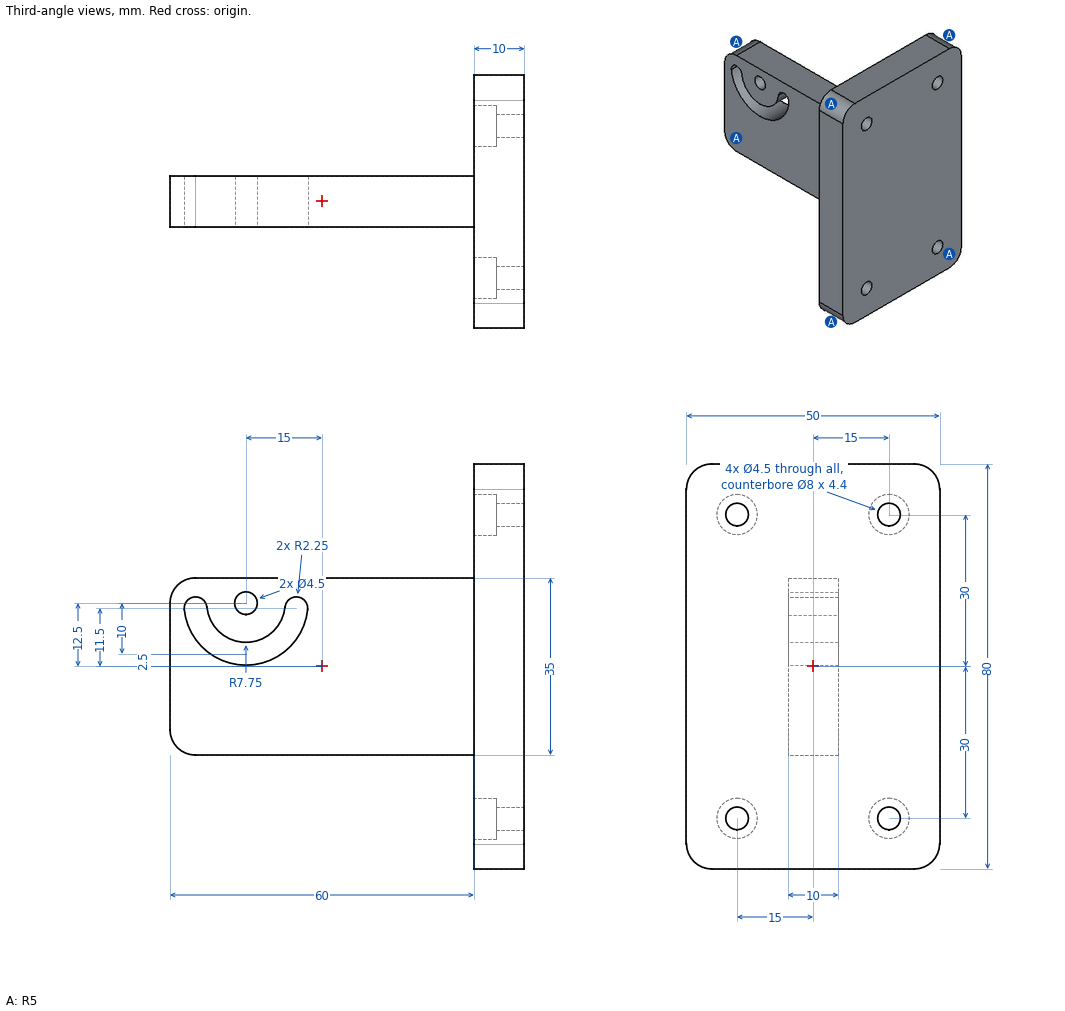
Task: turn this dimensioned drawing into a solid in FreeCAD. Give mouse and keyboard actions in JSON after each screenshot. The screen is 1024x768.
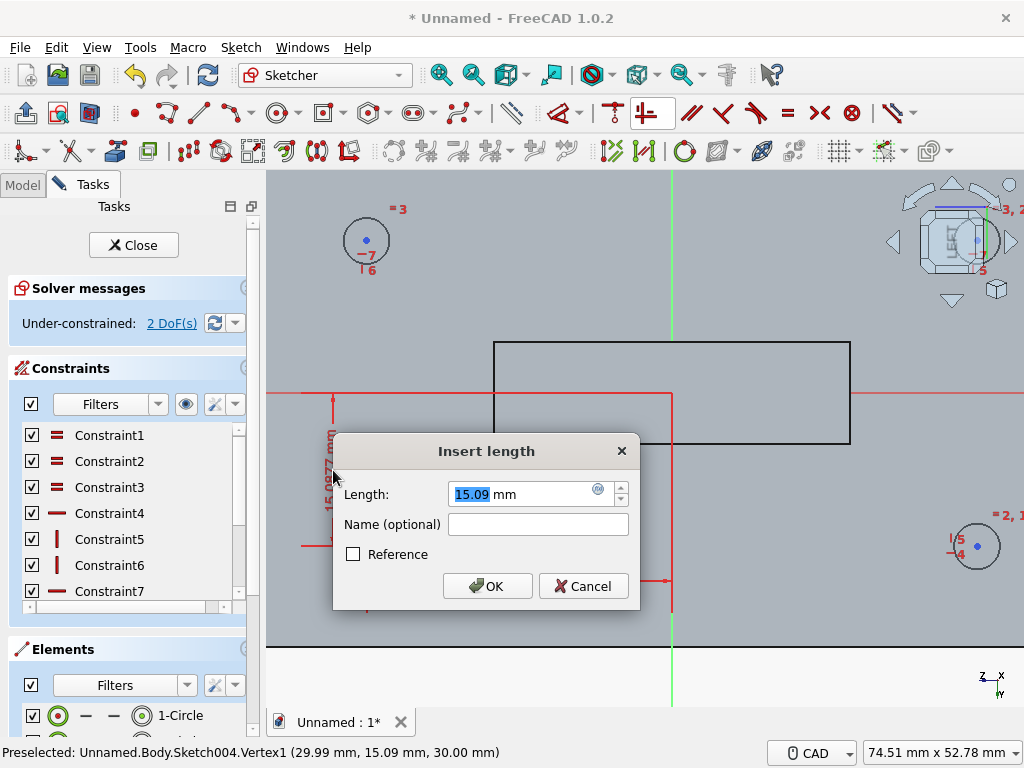
{"action": "type", "text": "15"}
{"action": "key", "text": "Return"}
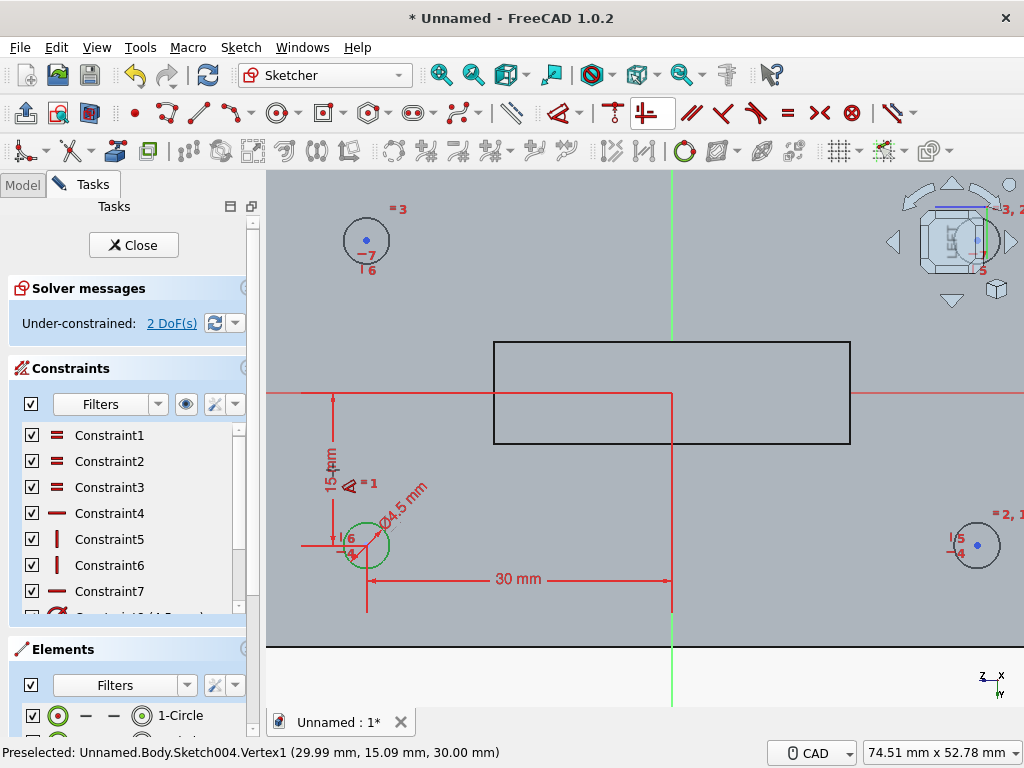
{"action": "scroll", "coordinate": [383, 531], "scroll_direction": "down", "scroll_amount": 2}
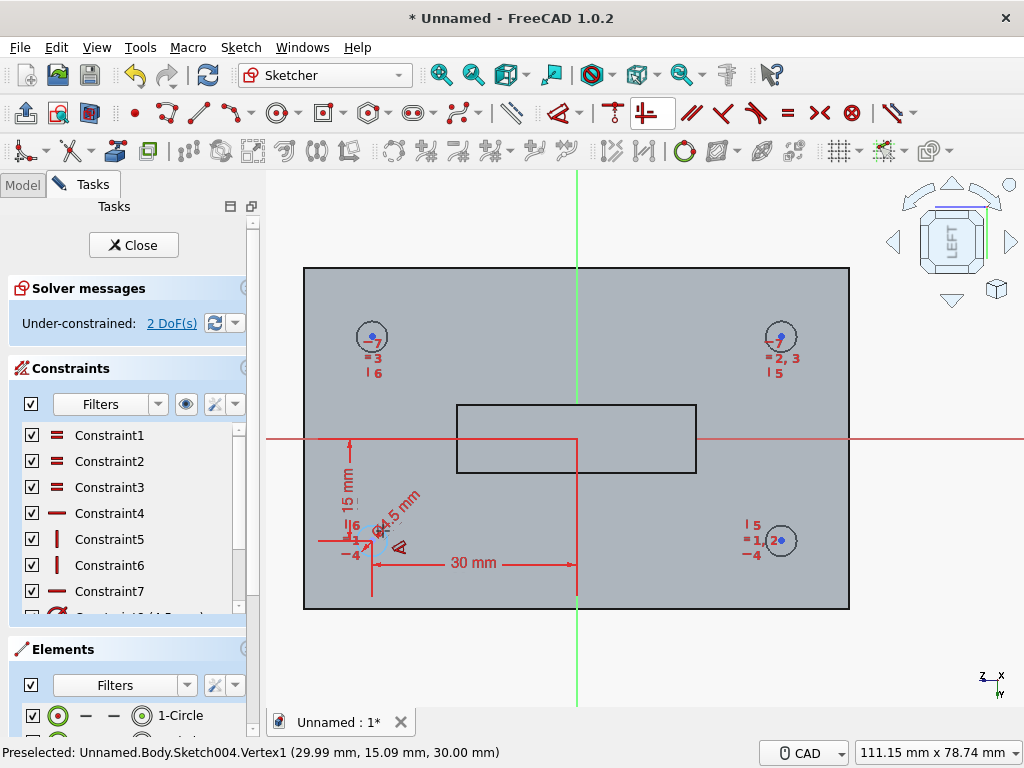
{"action": "left_click", "coordinate": [781, 541]}
{"action": "left_click", "coordinate": [679, 575]}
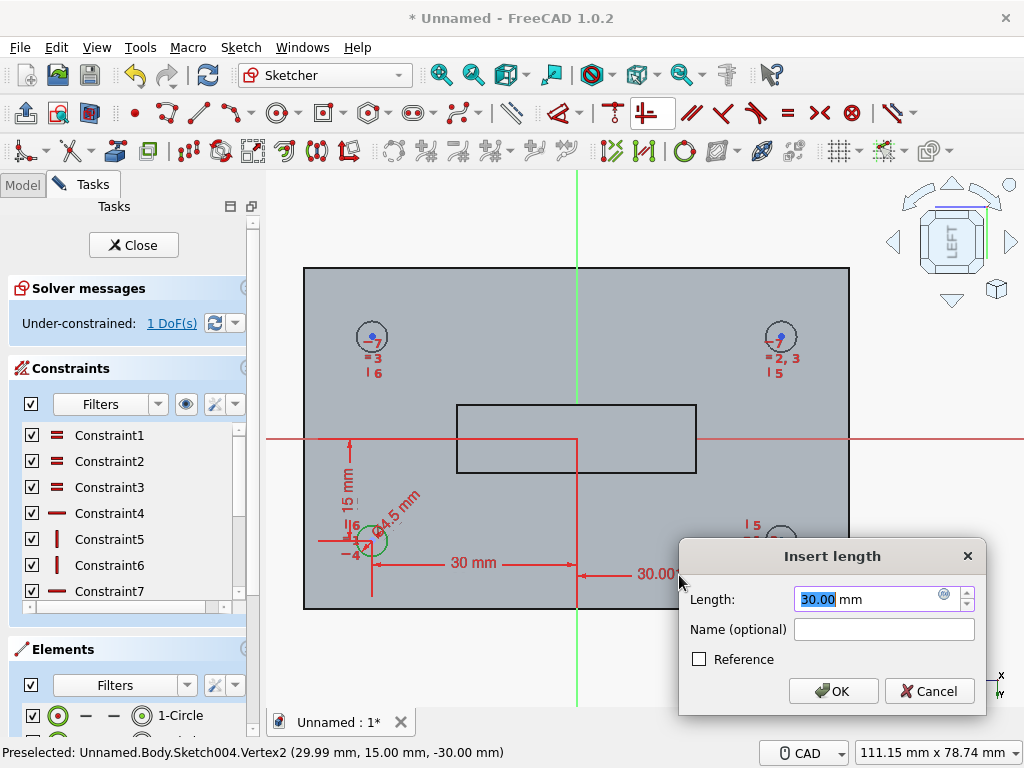
{"action": "type", "text": "30"}
{"action": "key", "text": "Return"}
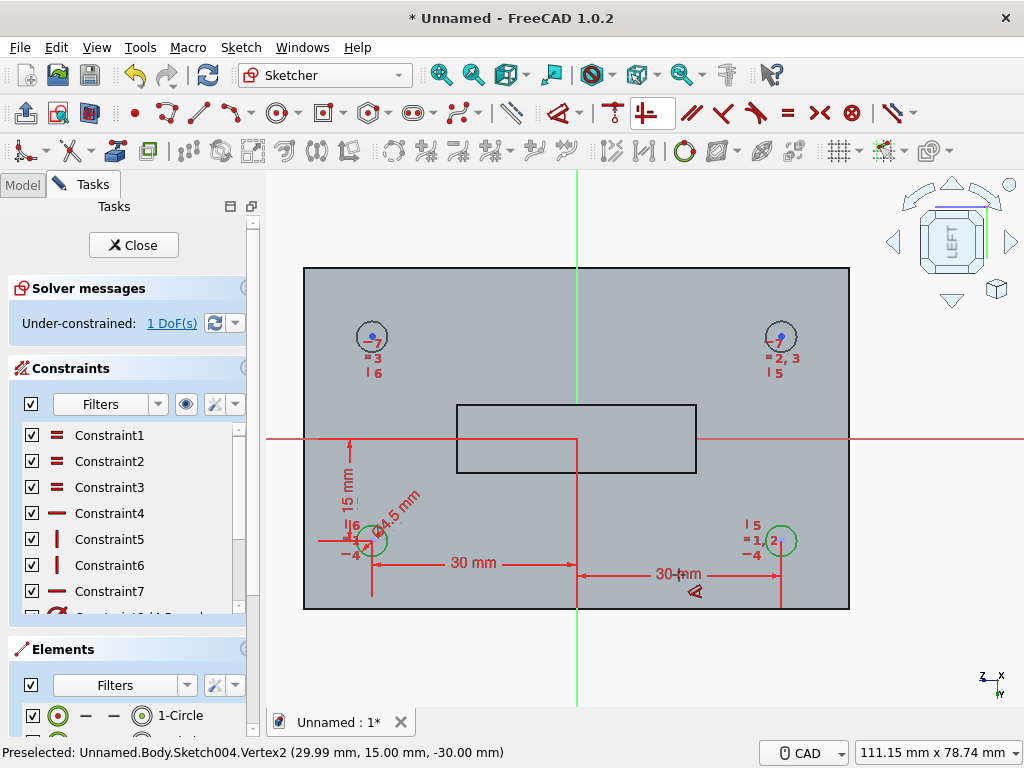
{"action": "left_click", "coordinate": [781, 337]}
{"action": "left_click", "coordinate": [815, 388]}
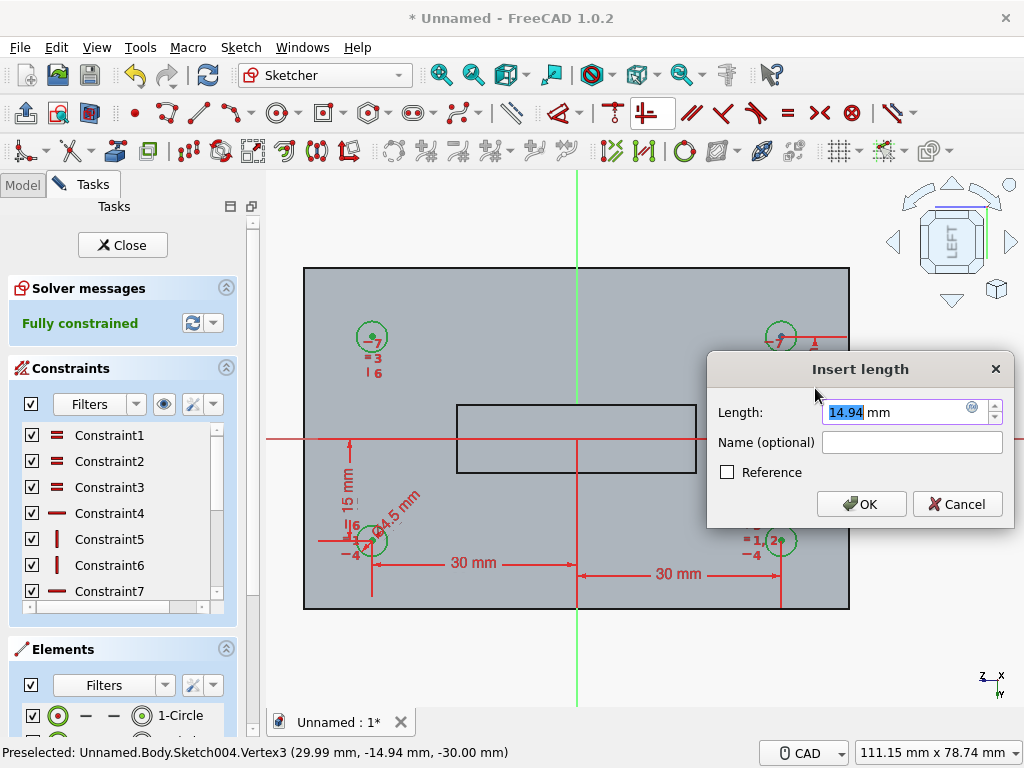
{"action": "type", "text": "15"}
{"action": "key", "text": "Return"}
{"action": "key", "text": "Escape"}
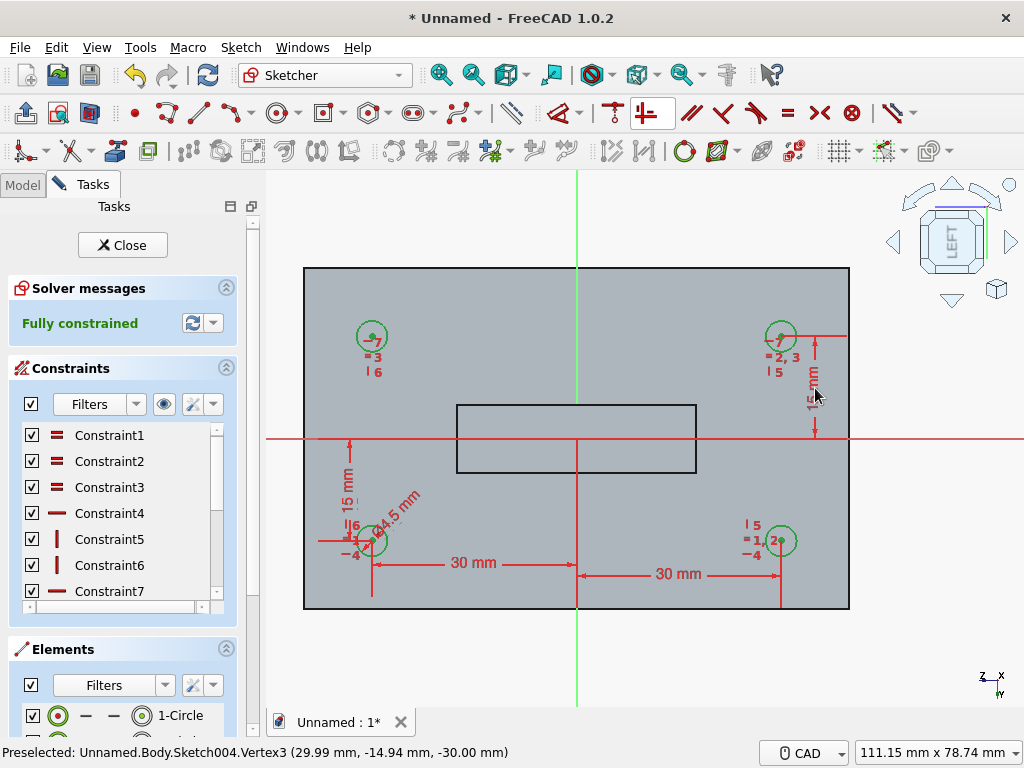
{"action": "left_click", "coordinate": [123, 245]}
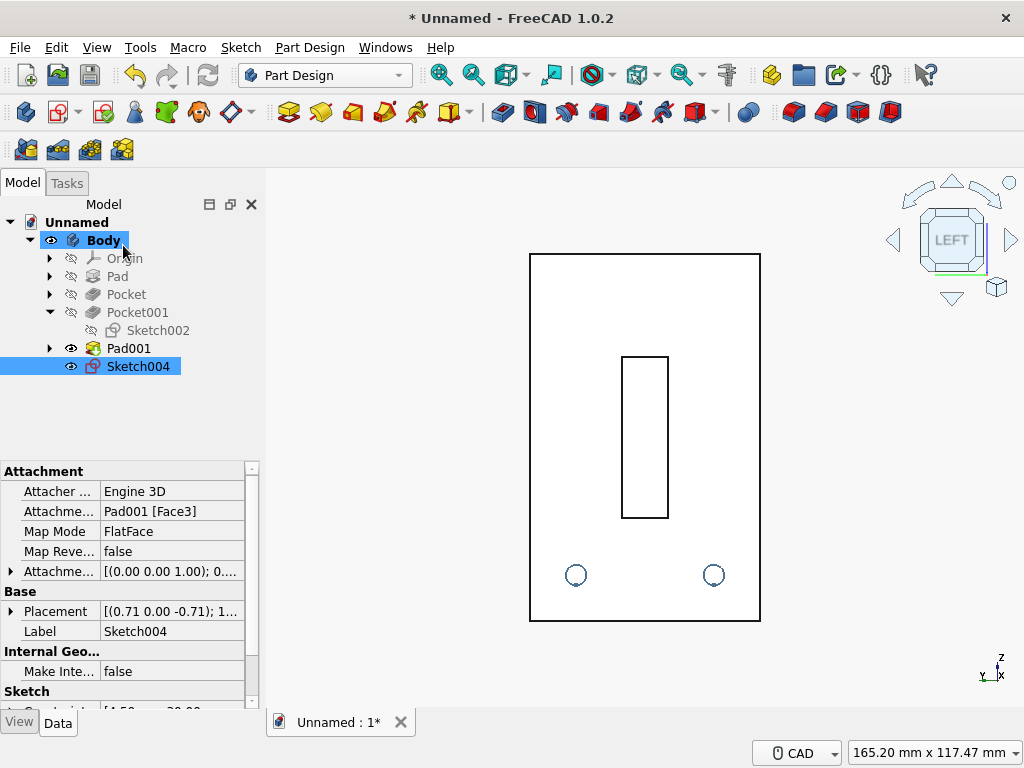
{"action": "left_click", "coordinate": [536, 112]}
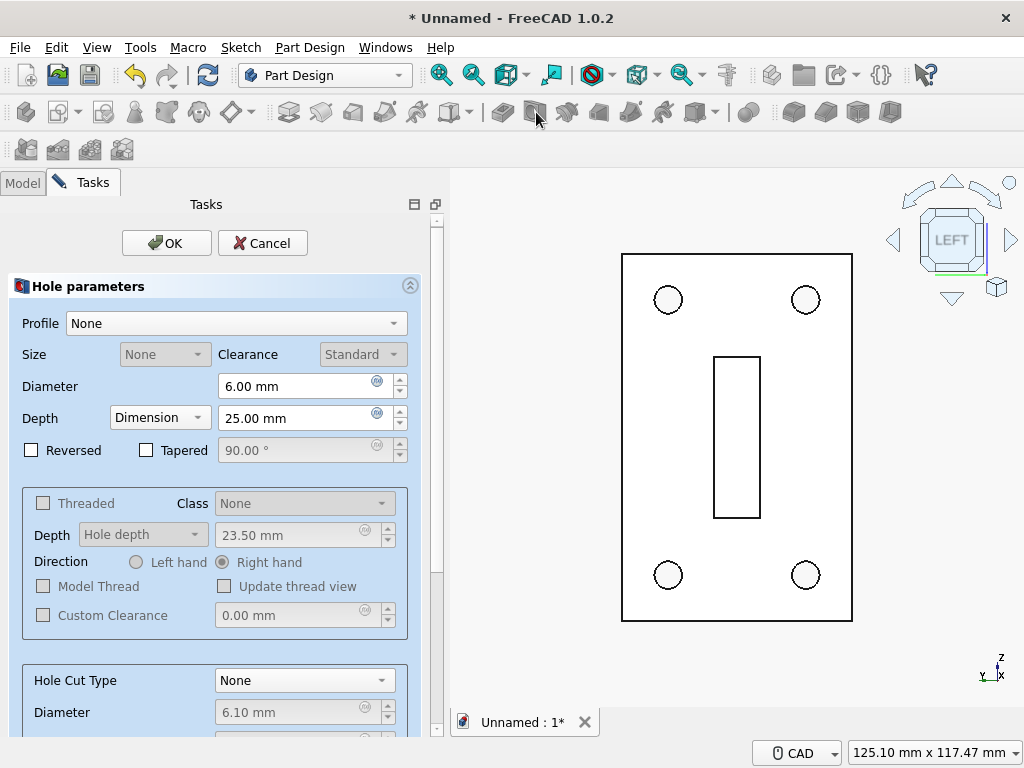
{"action": "triple_click", "coordinate": [305, 386]}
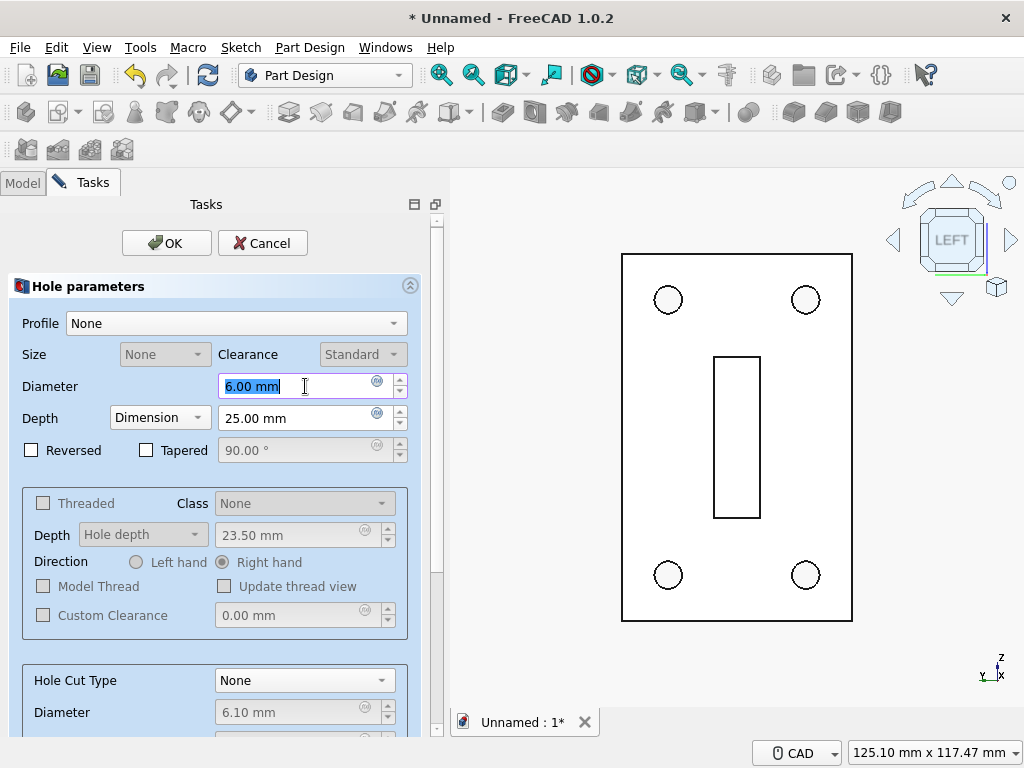
{"action": "type", "text": "4.5"}
{"action": "key", "text": "Tab"}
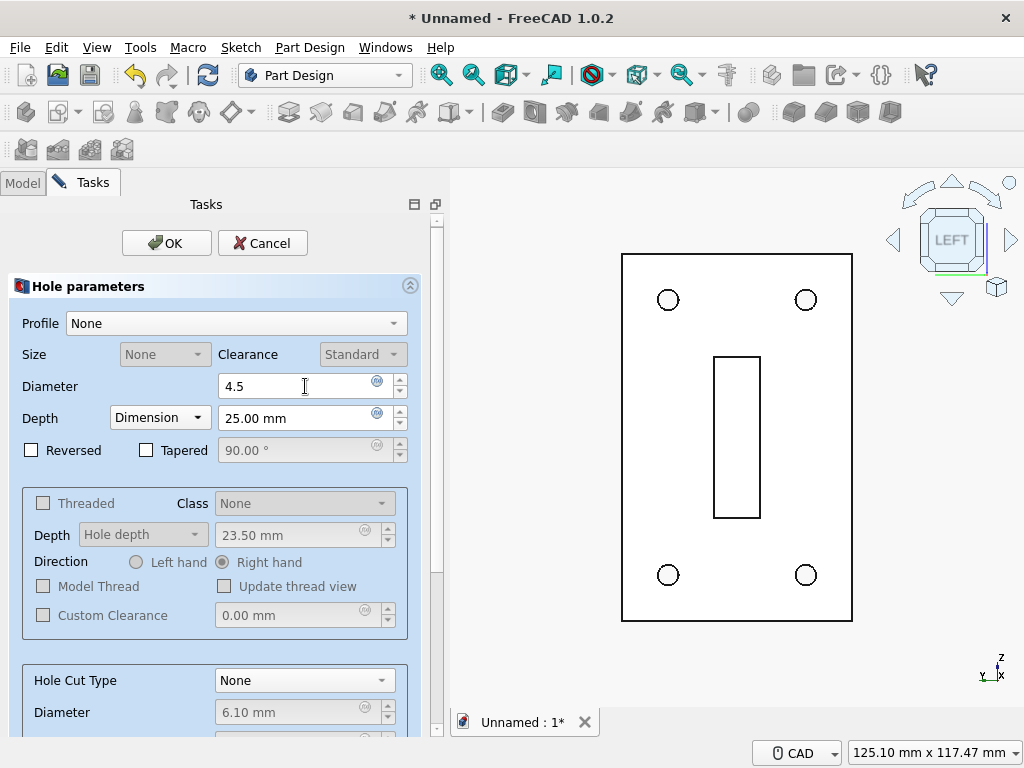
{"action": "left_click", "coordinate": [161, 418]}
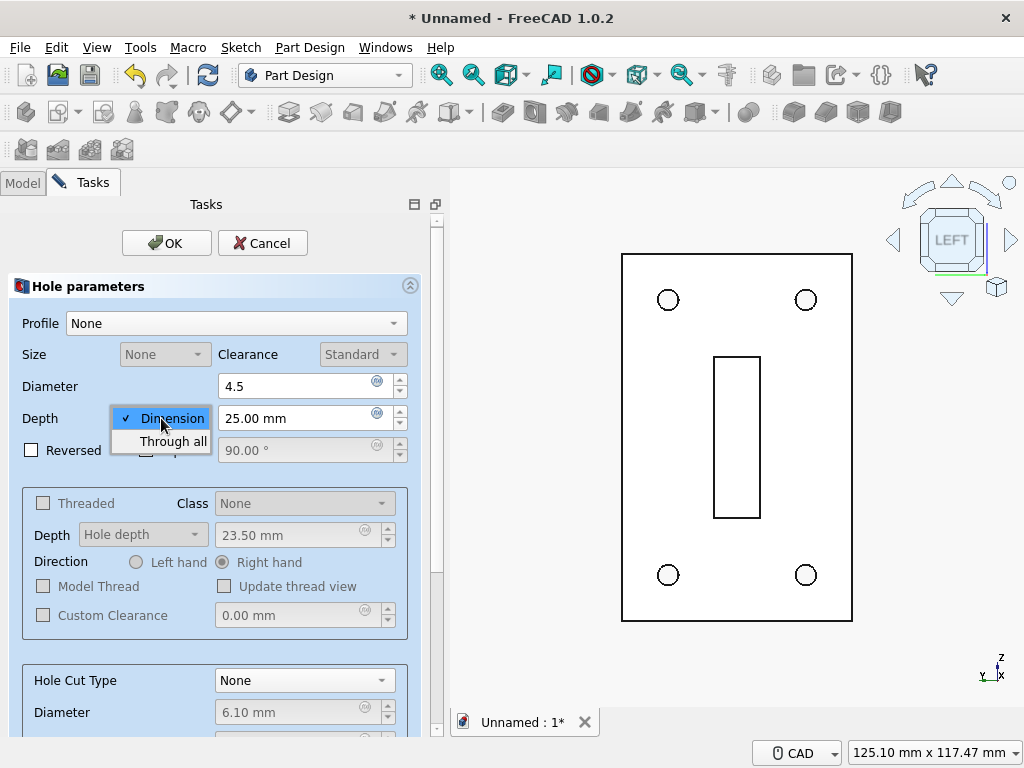
{"action": "left_click", "coordinate": [160, 442]}